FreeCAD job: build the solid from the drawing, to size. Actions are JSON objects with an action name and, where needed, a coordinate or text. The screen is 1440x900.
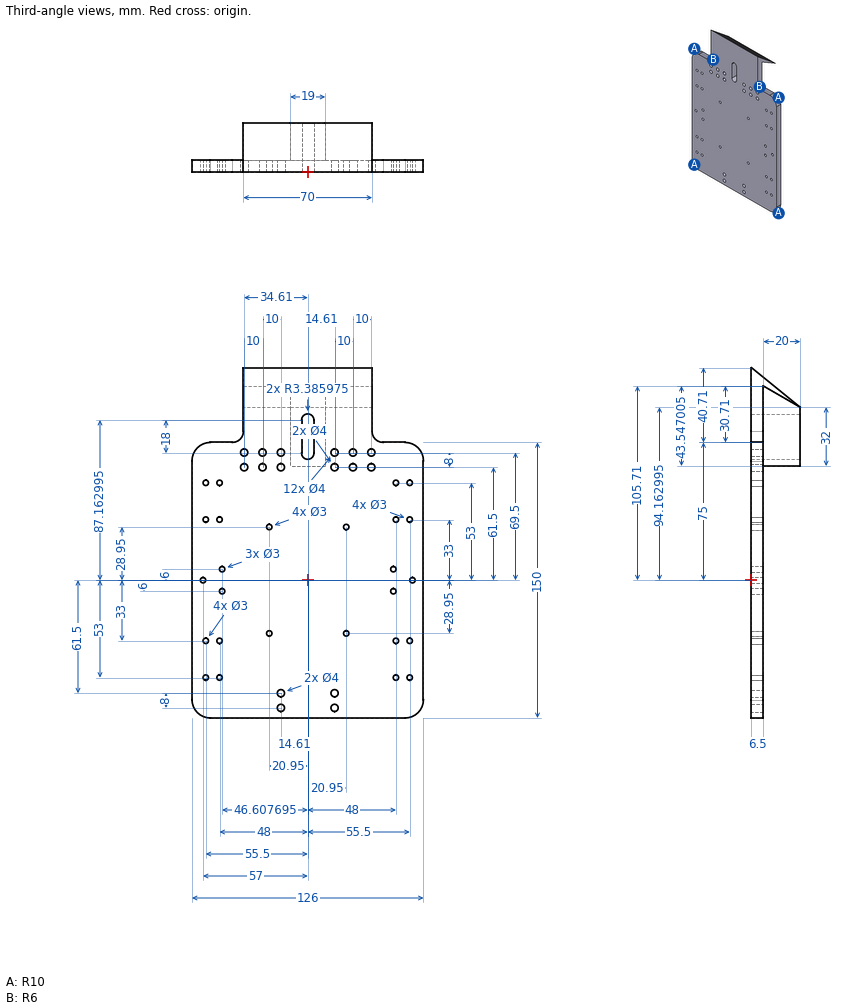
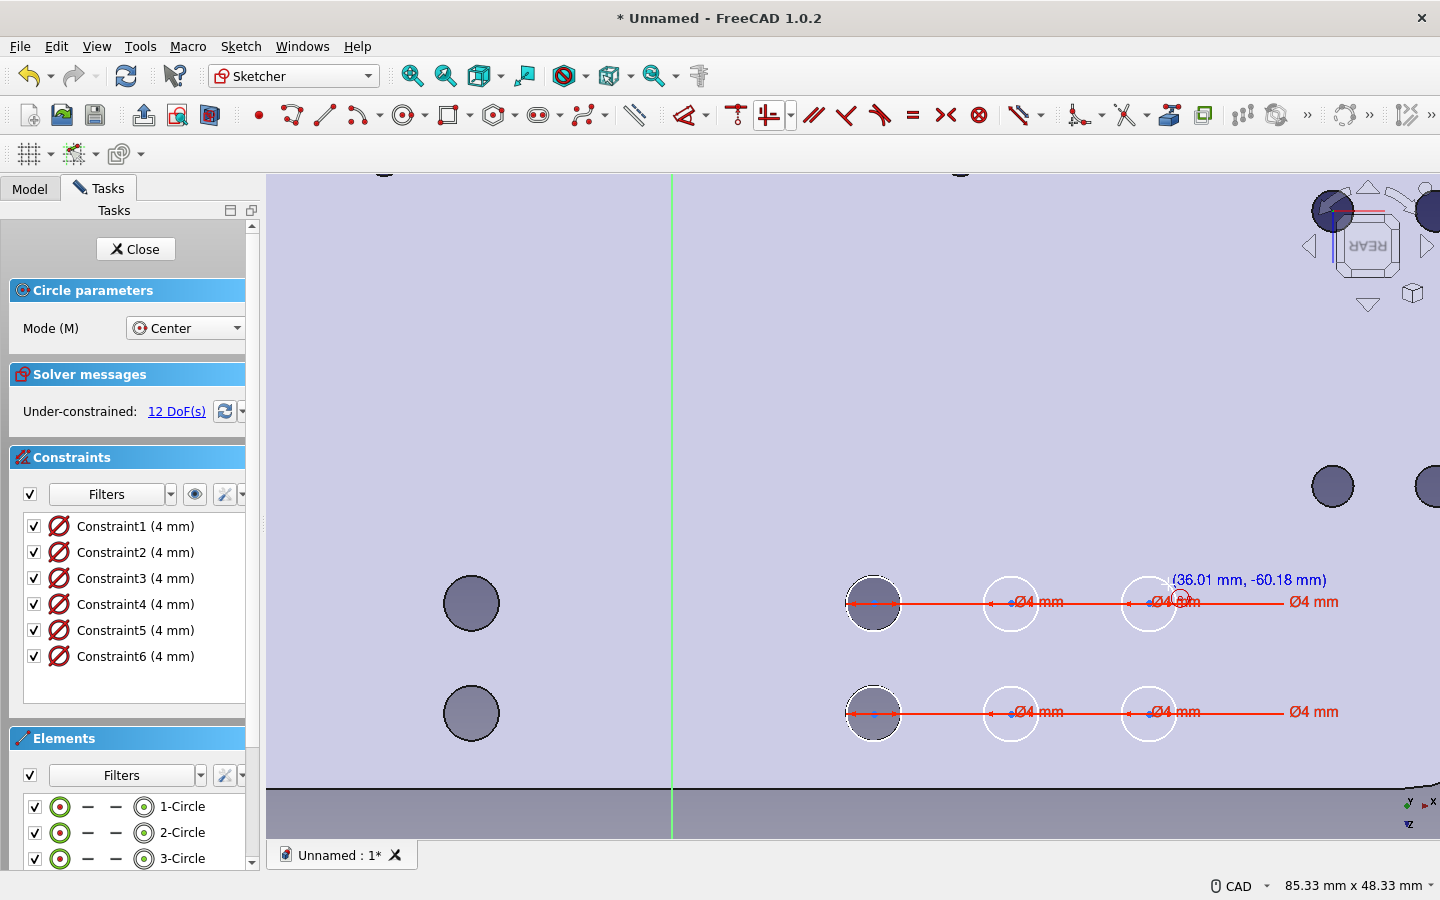
{"action": "scroll", "coordinate": [876, 717], "scroll_direction": "down", "scroll_amount": 4}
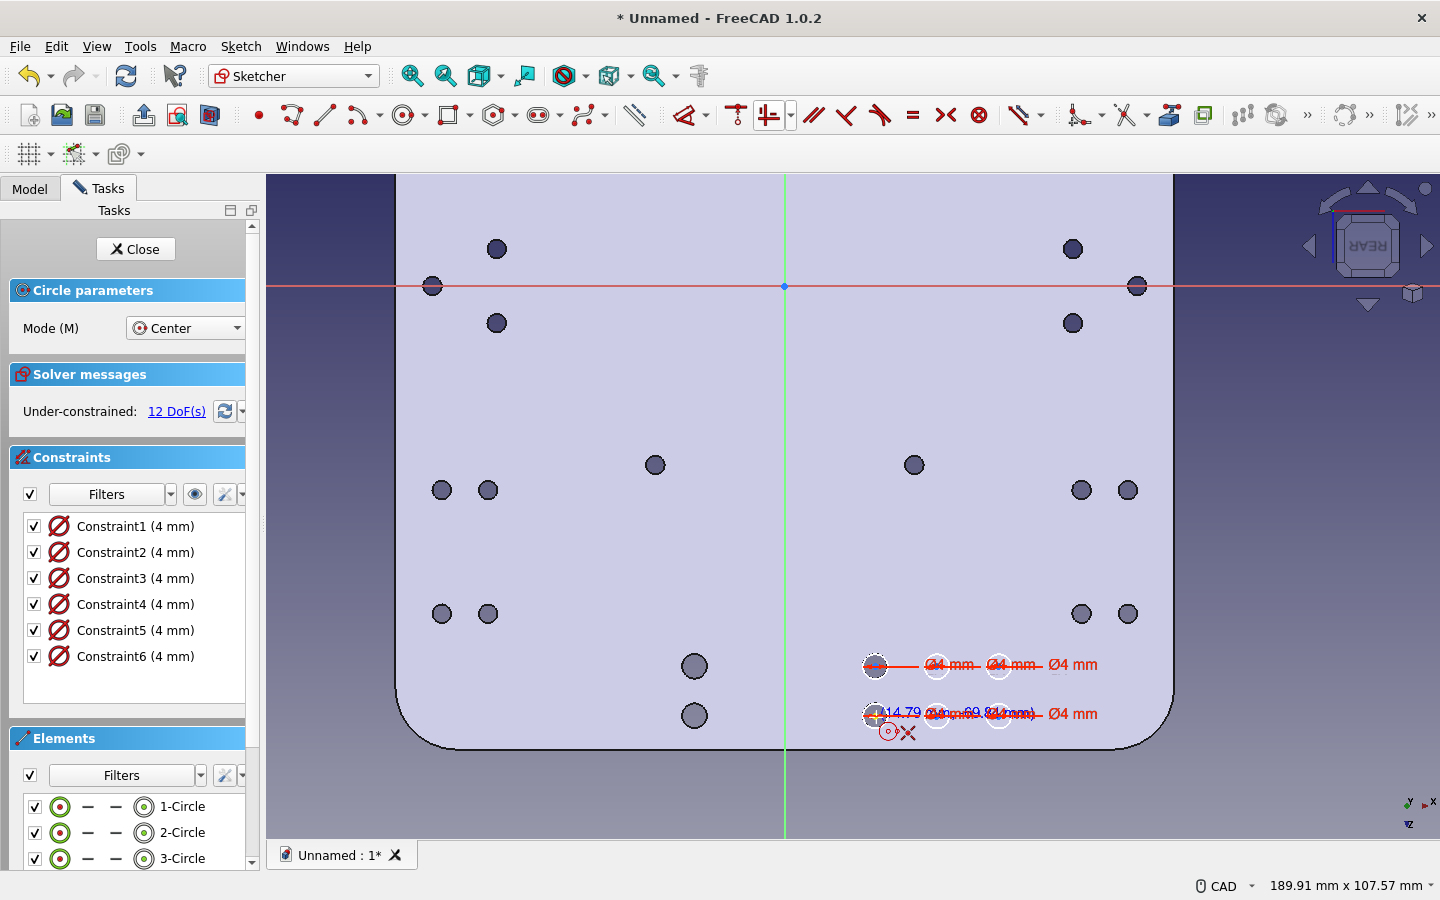
{"action": "scroll", "coordinate": [571, 666], "scroll_direction": "up", "scroll_amount": 4}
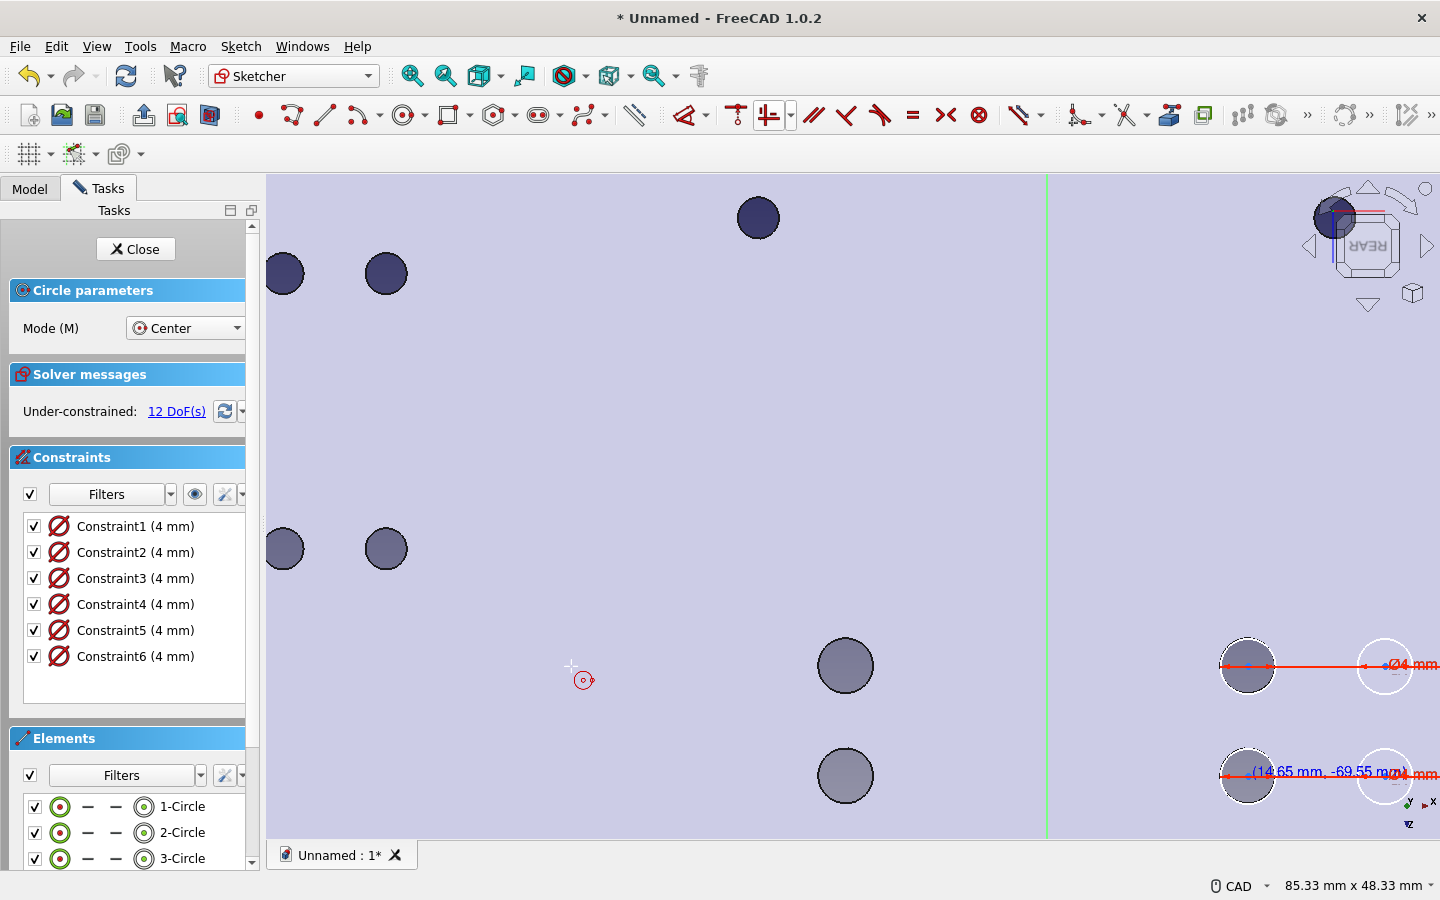
{"action": "left_click", "coordinate": [570, 666]}
{"action": "mouse_move", "coordinate": [590, 646]}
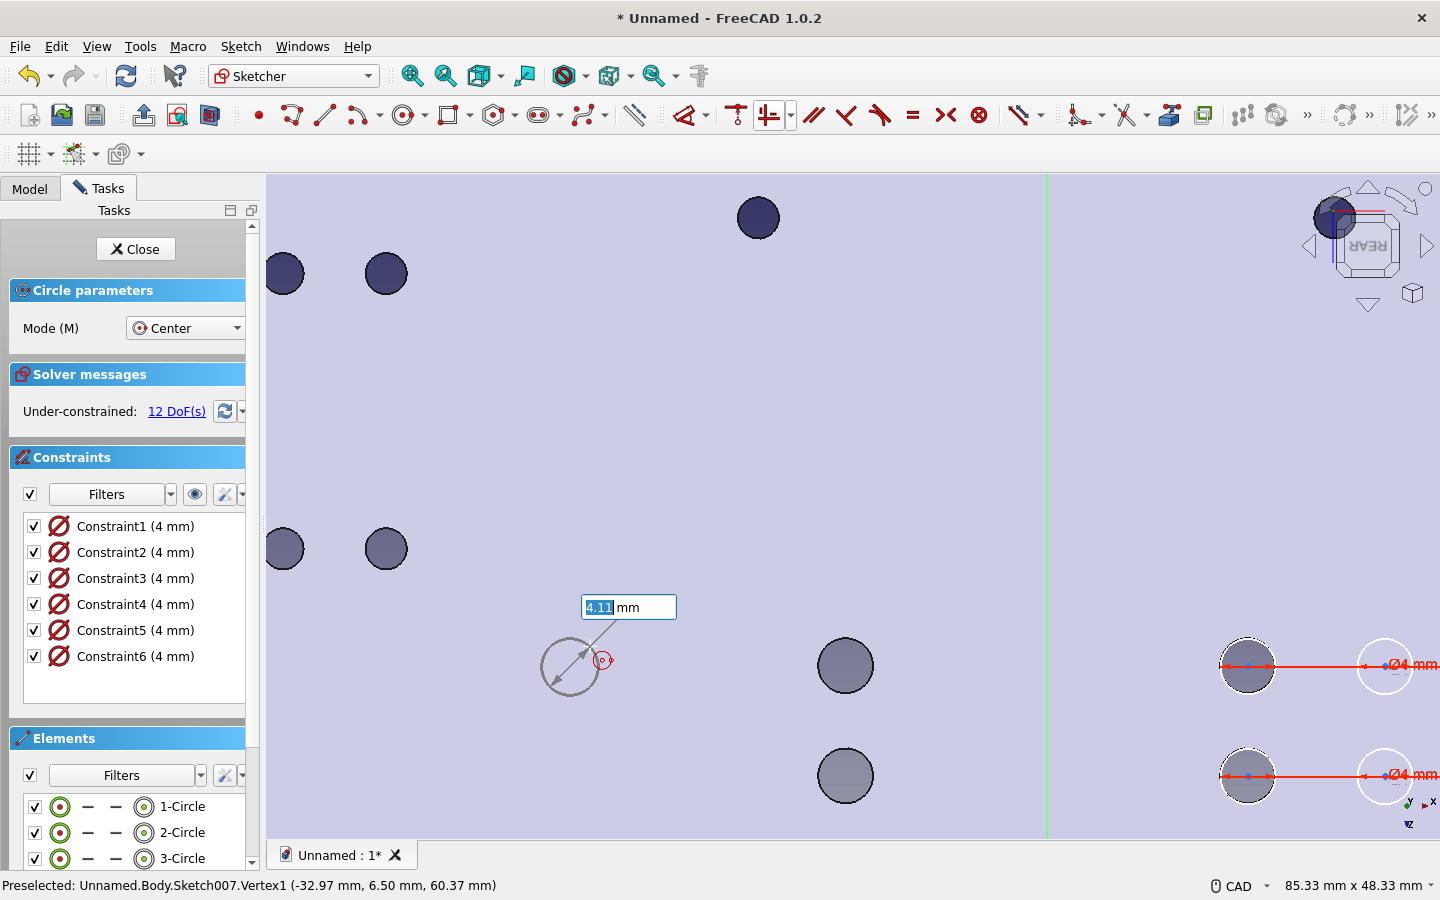
{"action": "type", "text": "4"}
{"action": "key", "text": "Return"}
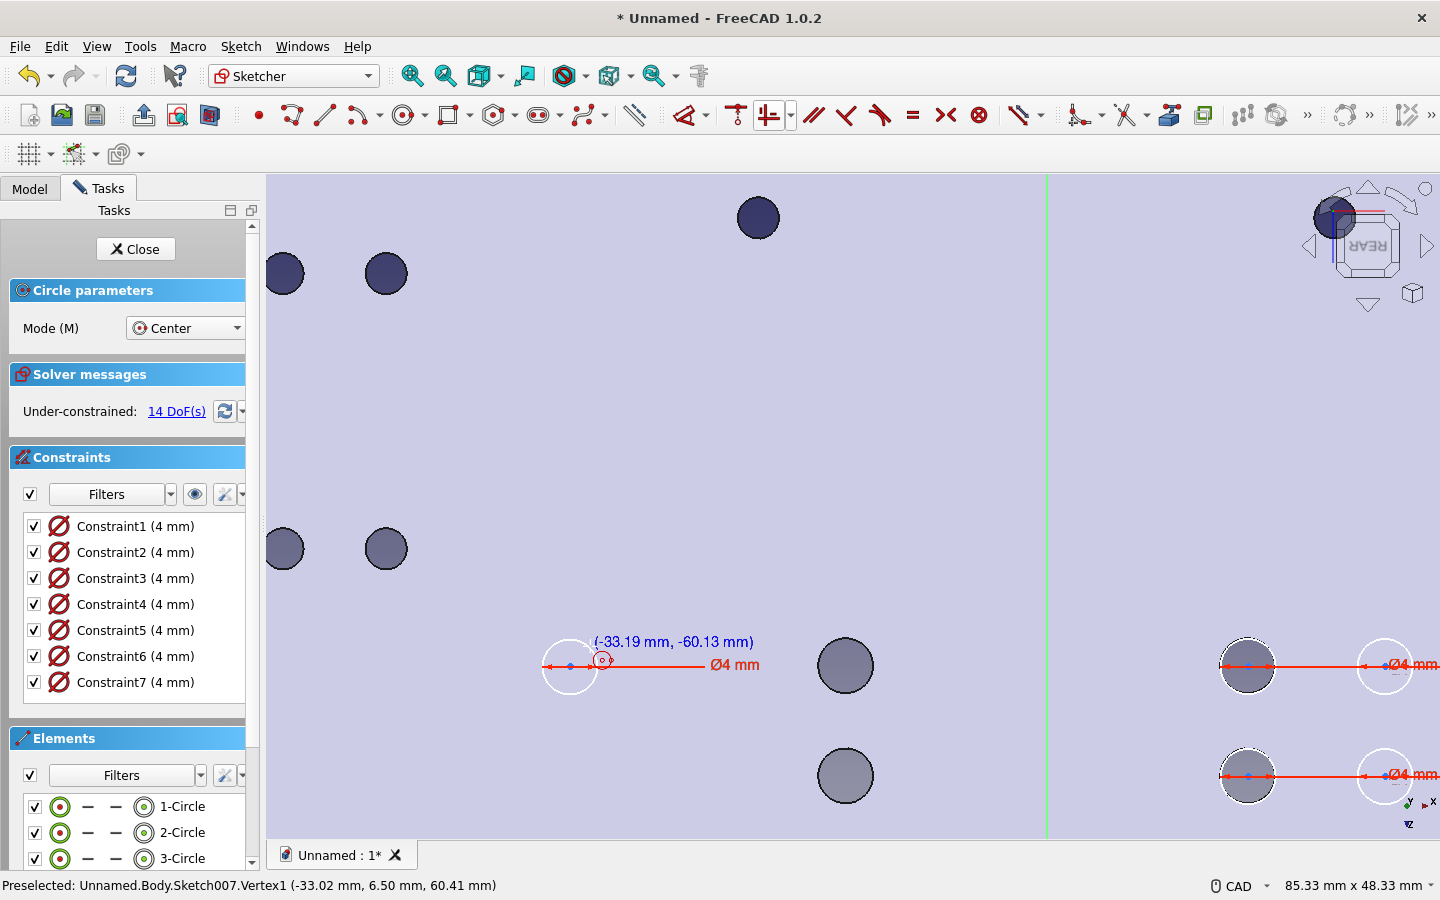
{"action": "left_click", "coordinate": [570, 776]}
{"action": "mouse_move", "coordinate": [590, 756]}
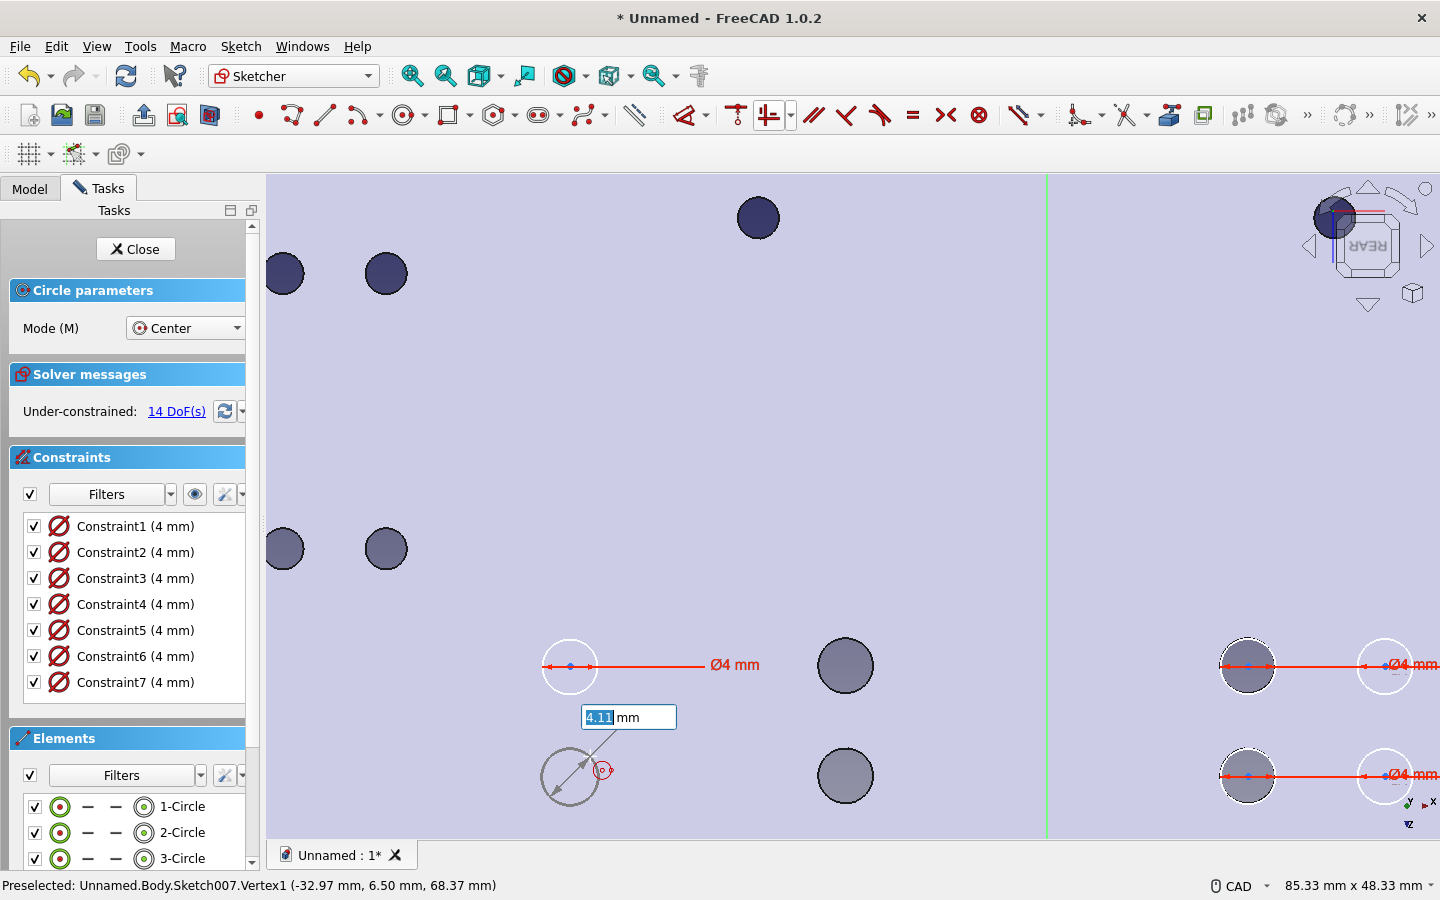
{"action": "type", "text": "4"}
{"action": "key", "text": "Return"}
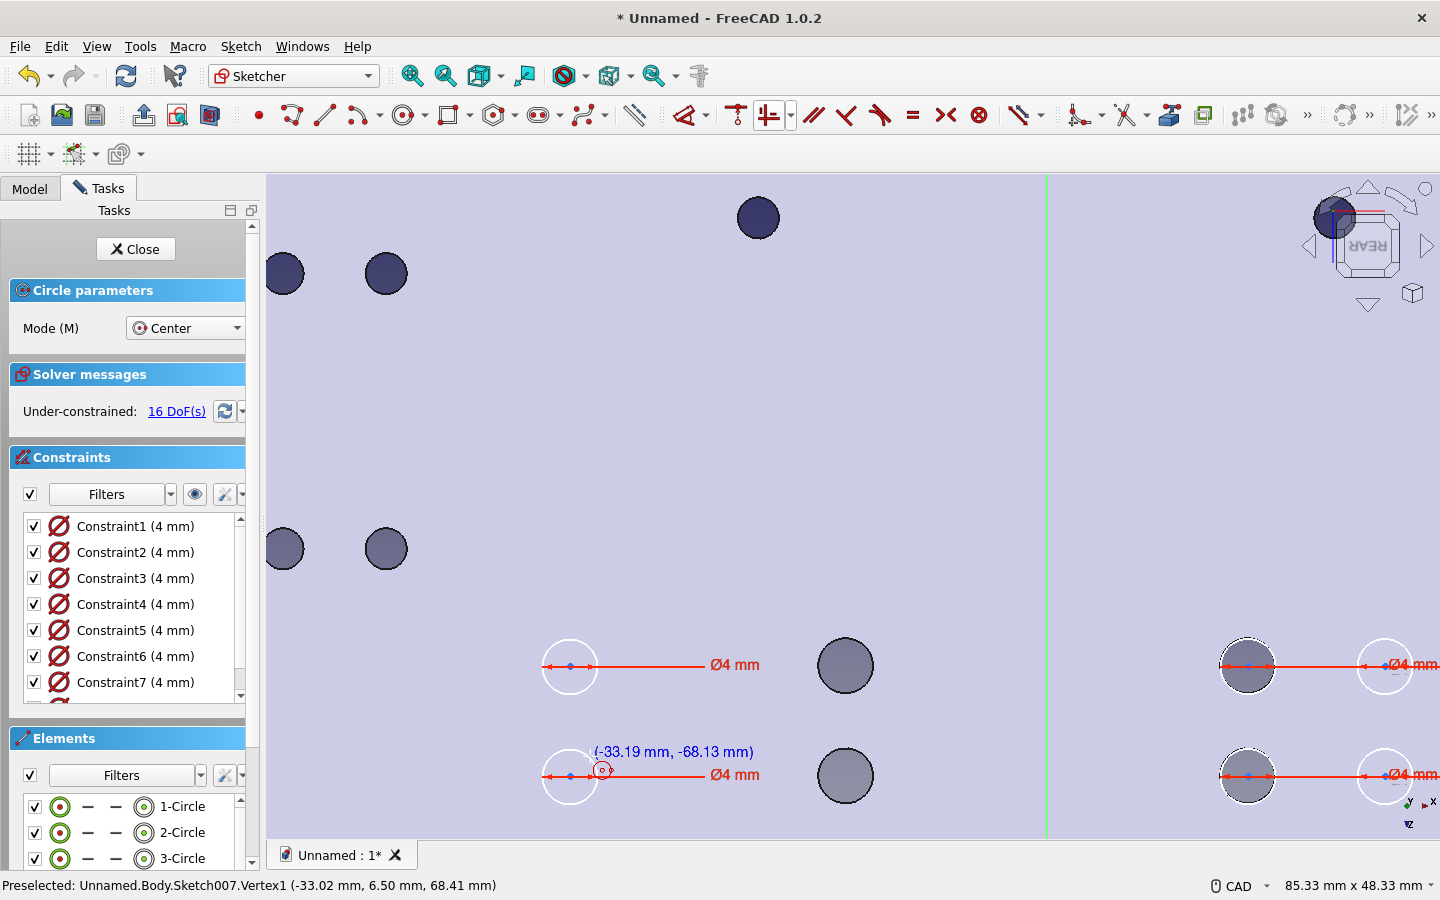
{"action": "left_click", "coordinate": [708, 666]}
{"action": "mouse_move", "coordinate": [727, 646]}